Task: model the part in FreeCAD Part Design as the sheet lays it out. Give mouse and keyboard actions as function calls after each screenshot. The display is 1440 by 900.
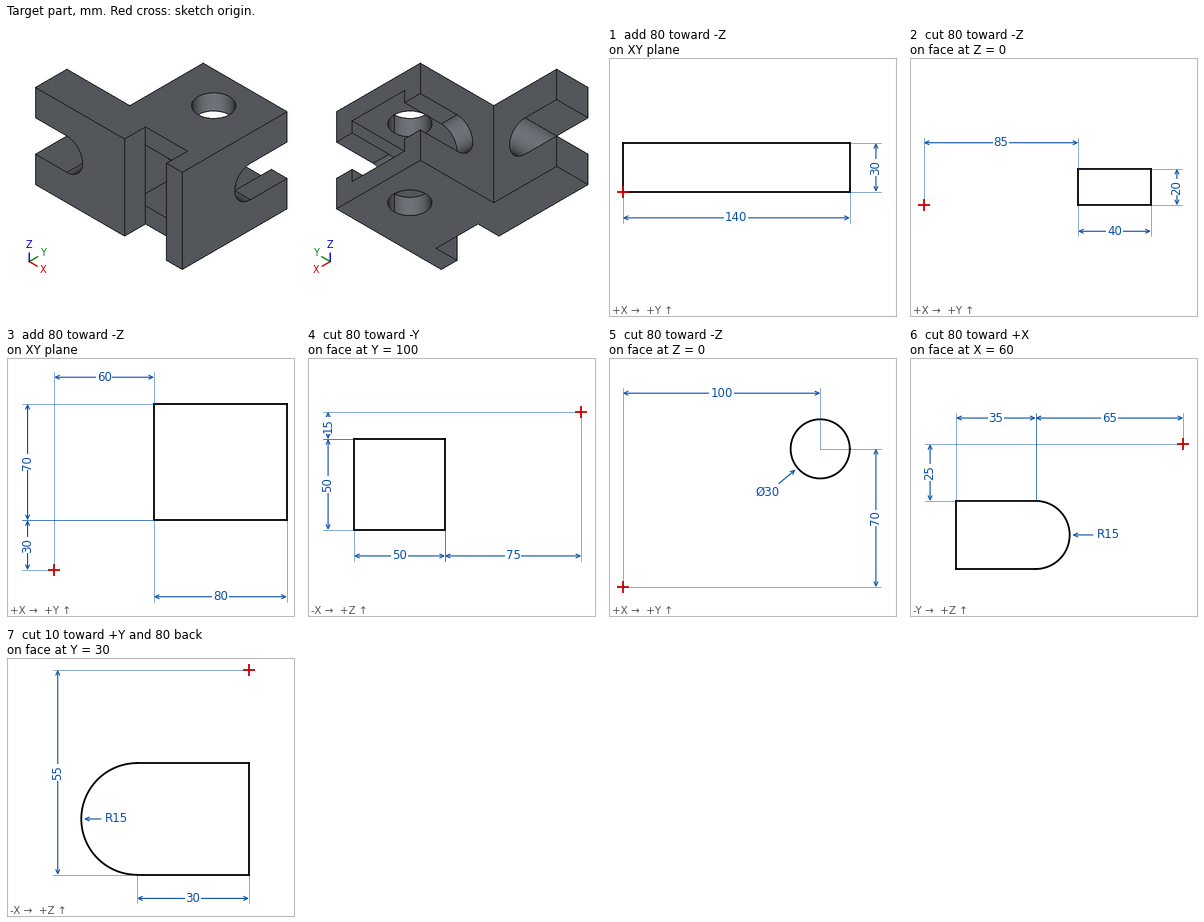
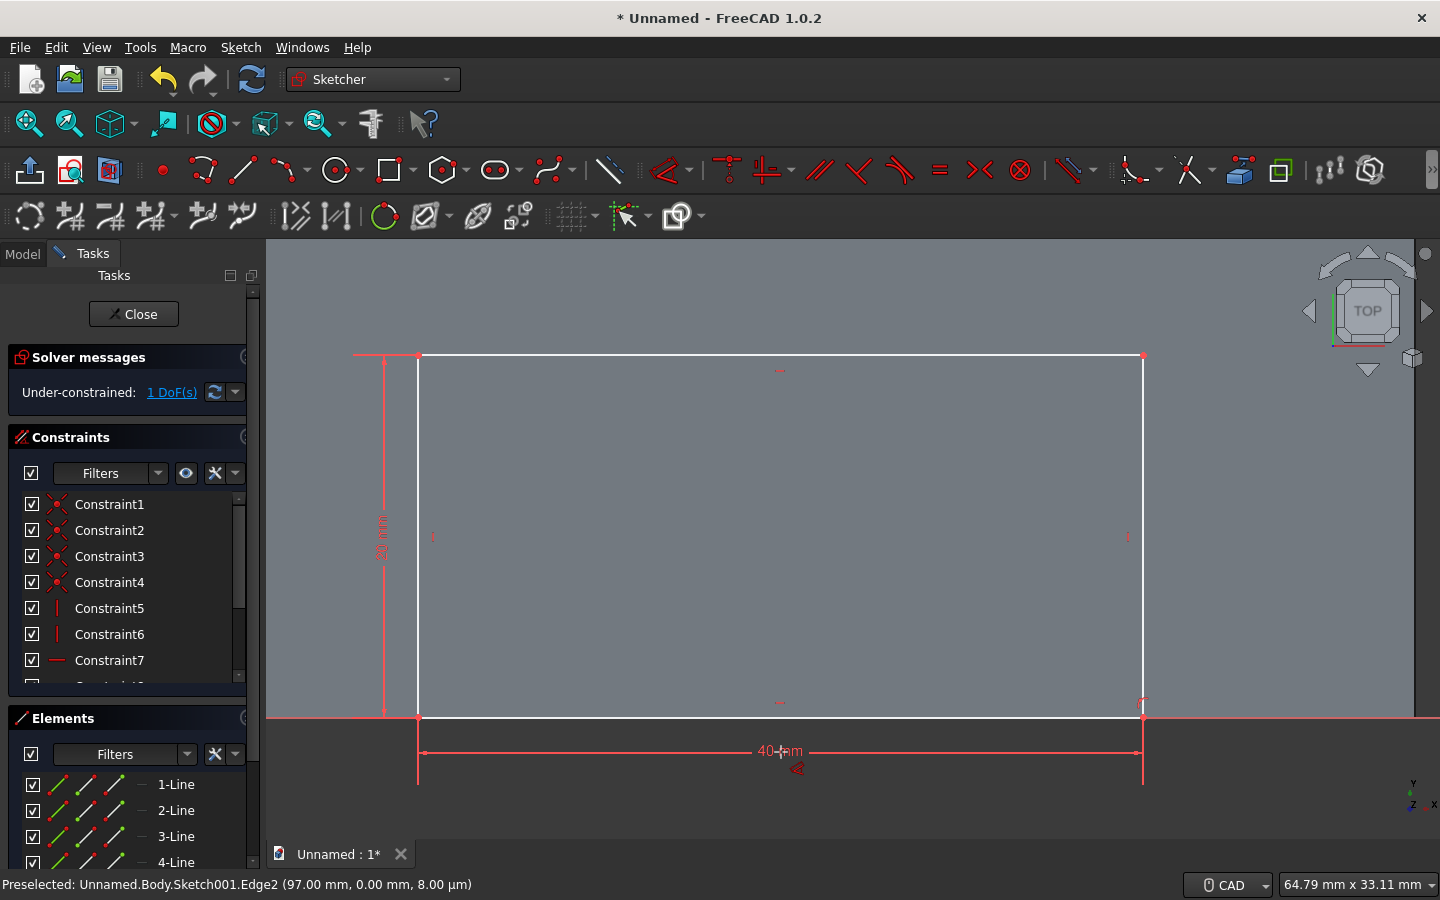
click(418, 355)
click(356, 752)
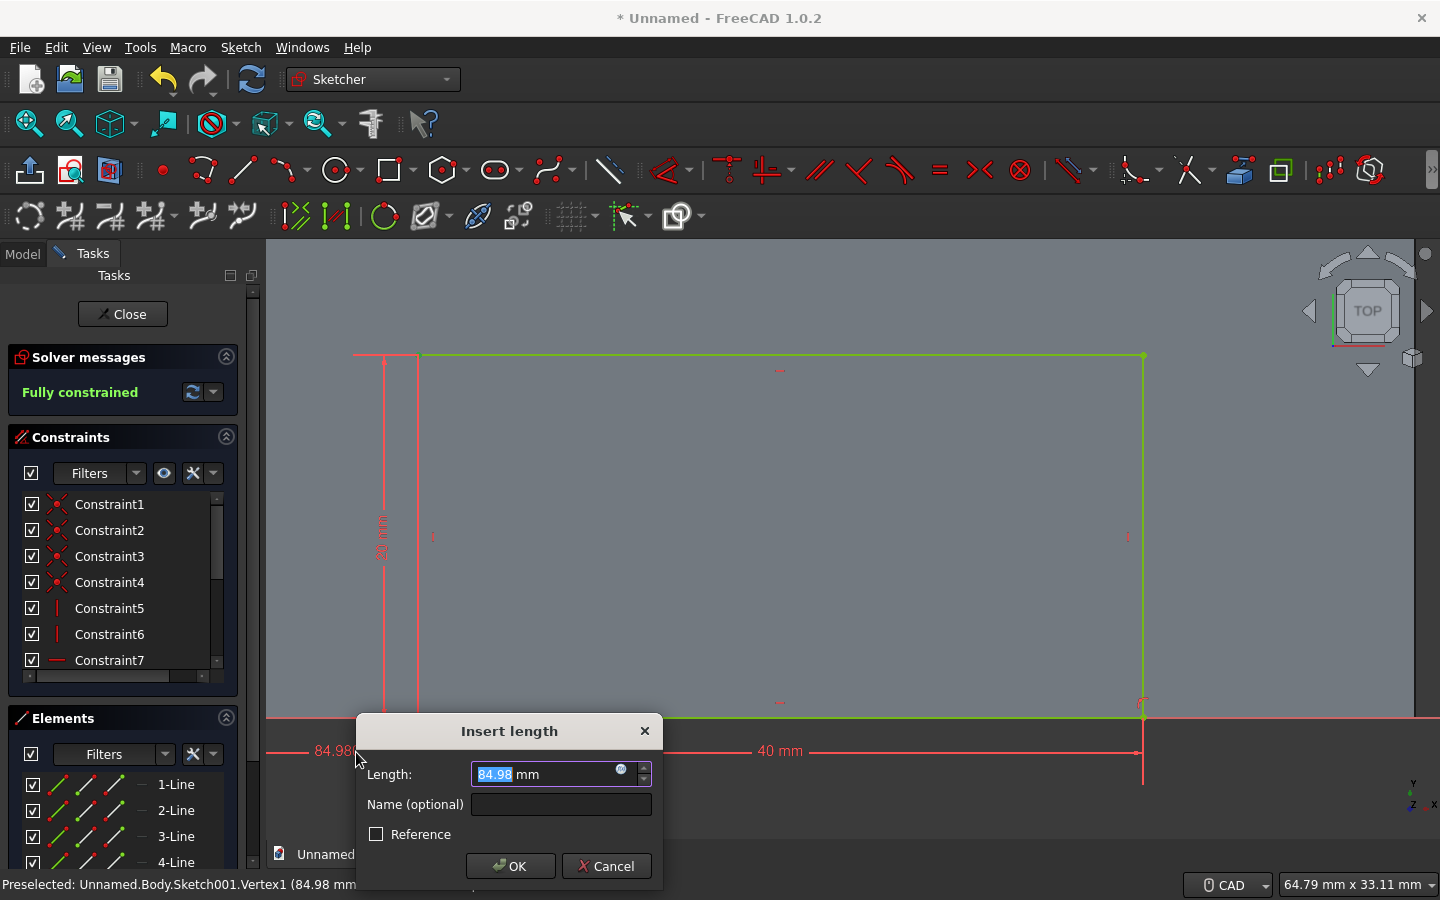
text(85)
key(Return)
key(Escape)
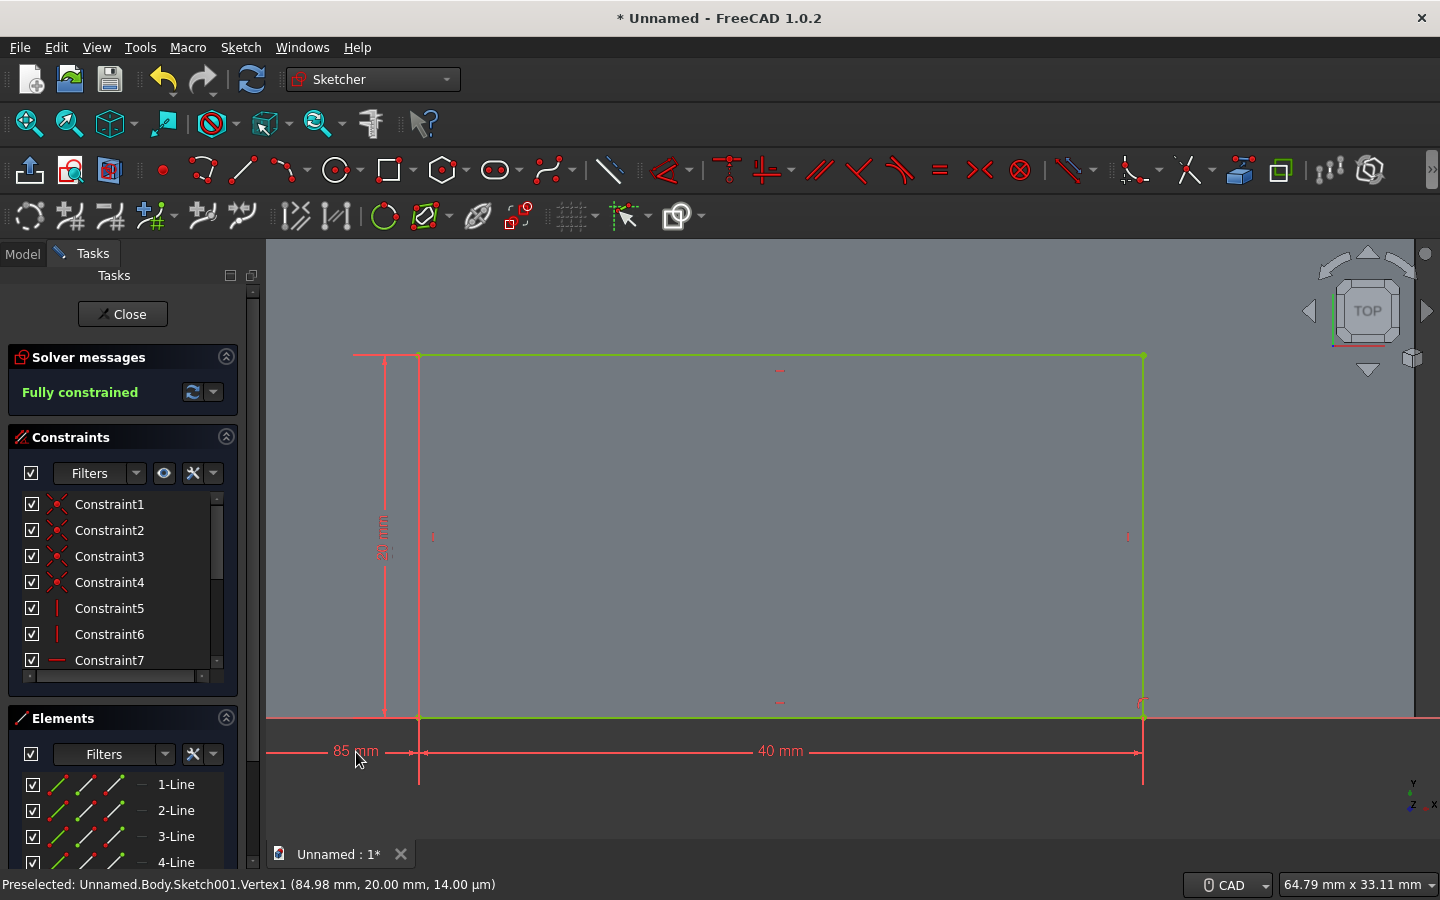
click(123, 314)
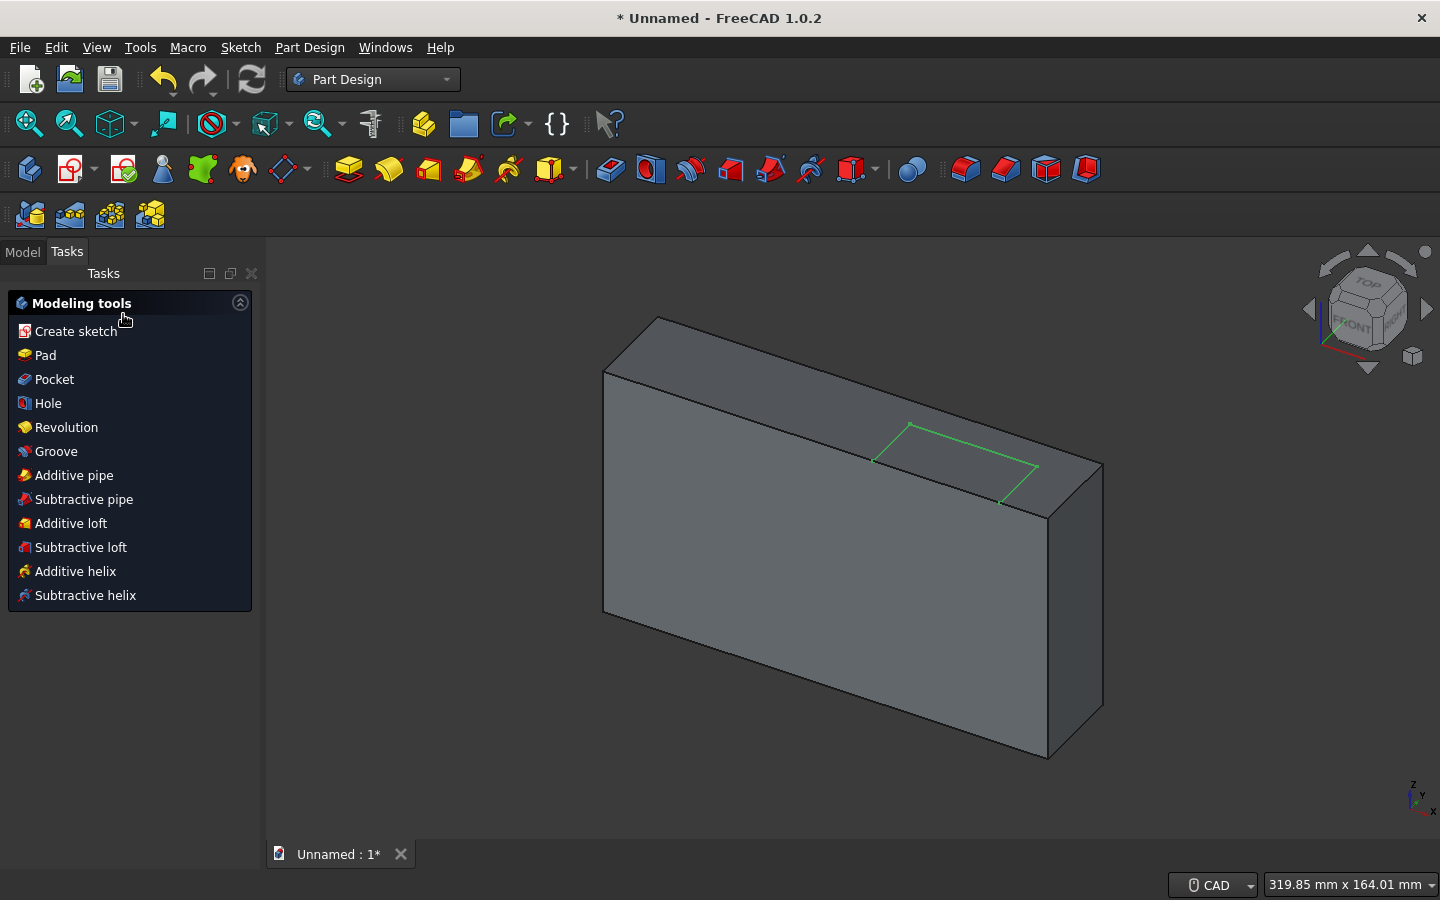
click(612, 170)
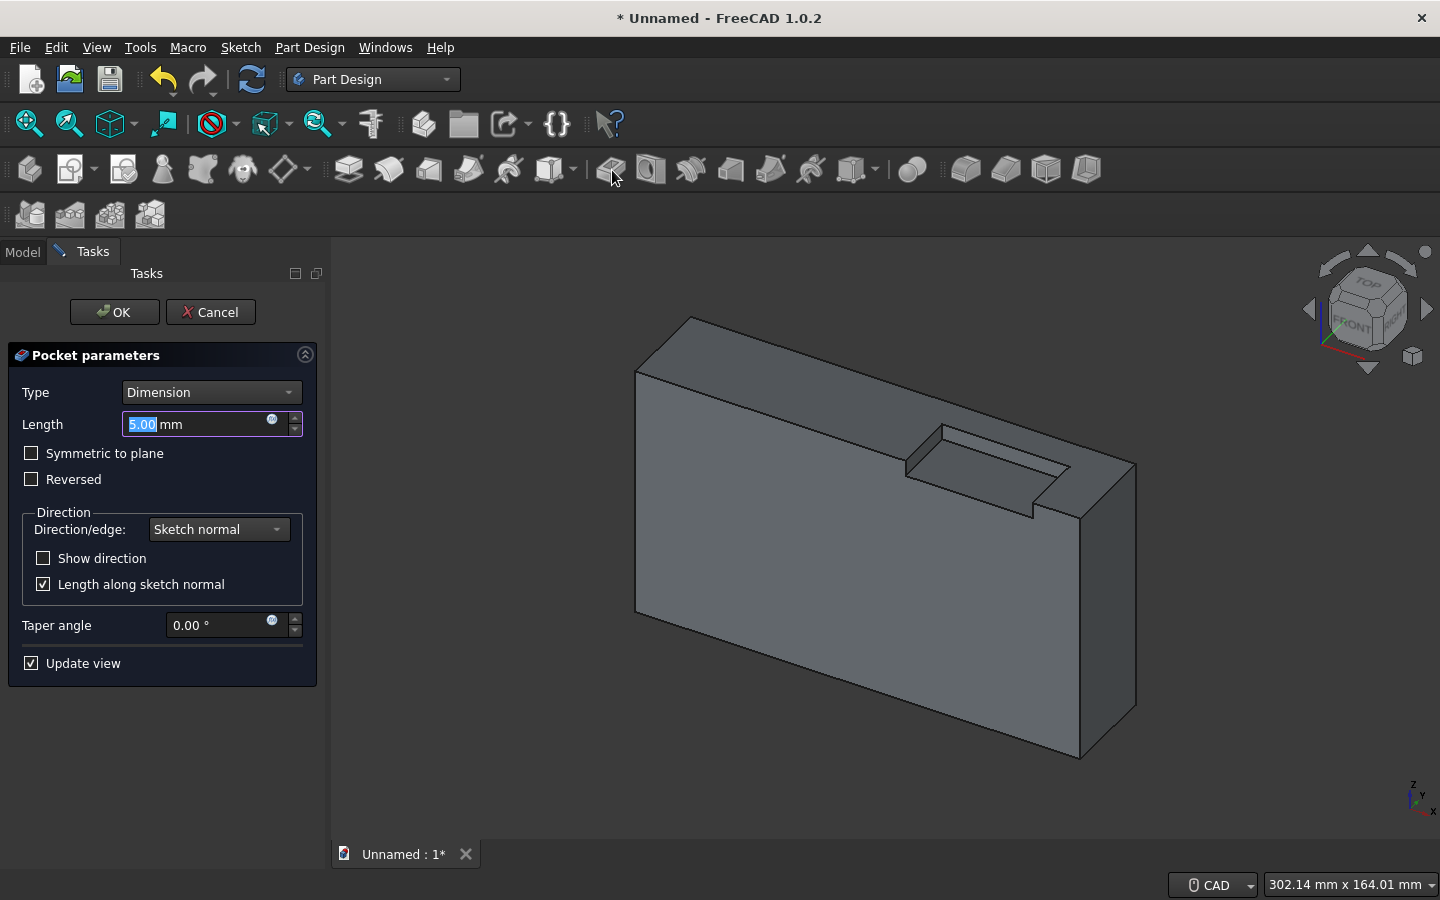
text(80)
key(Tab)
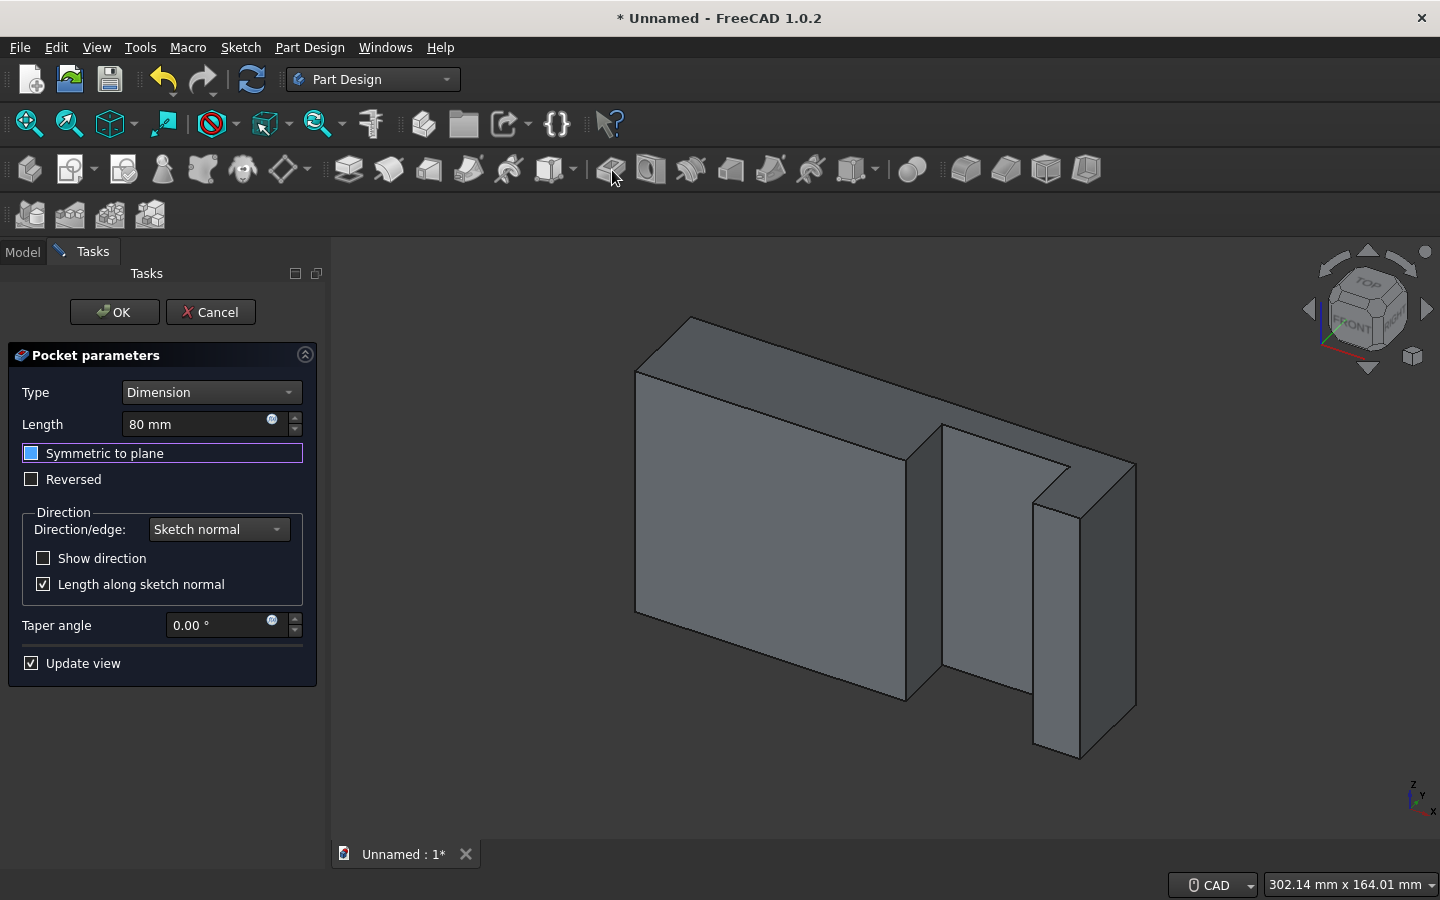
click(115, 312)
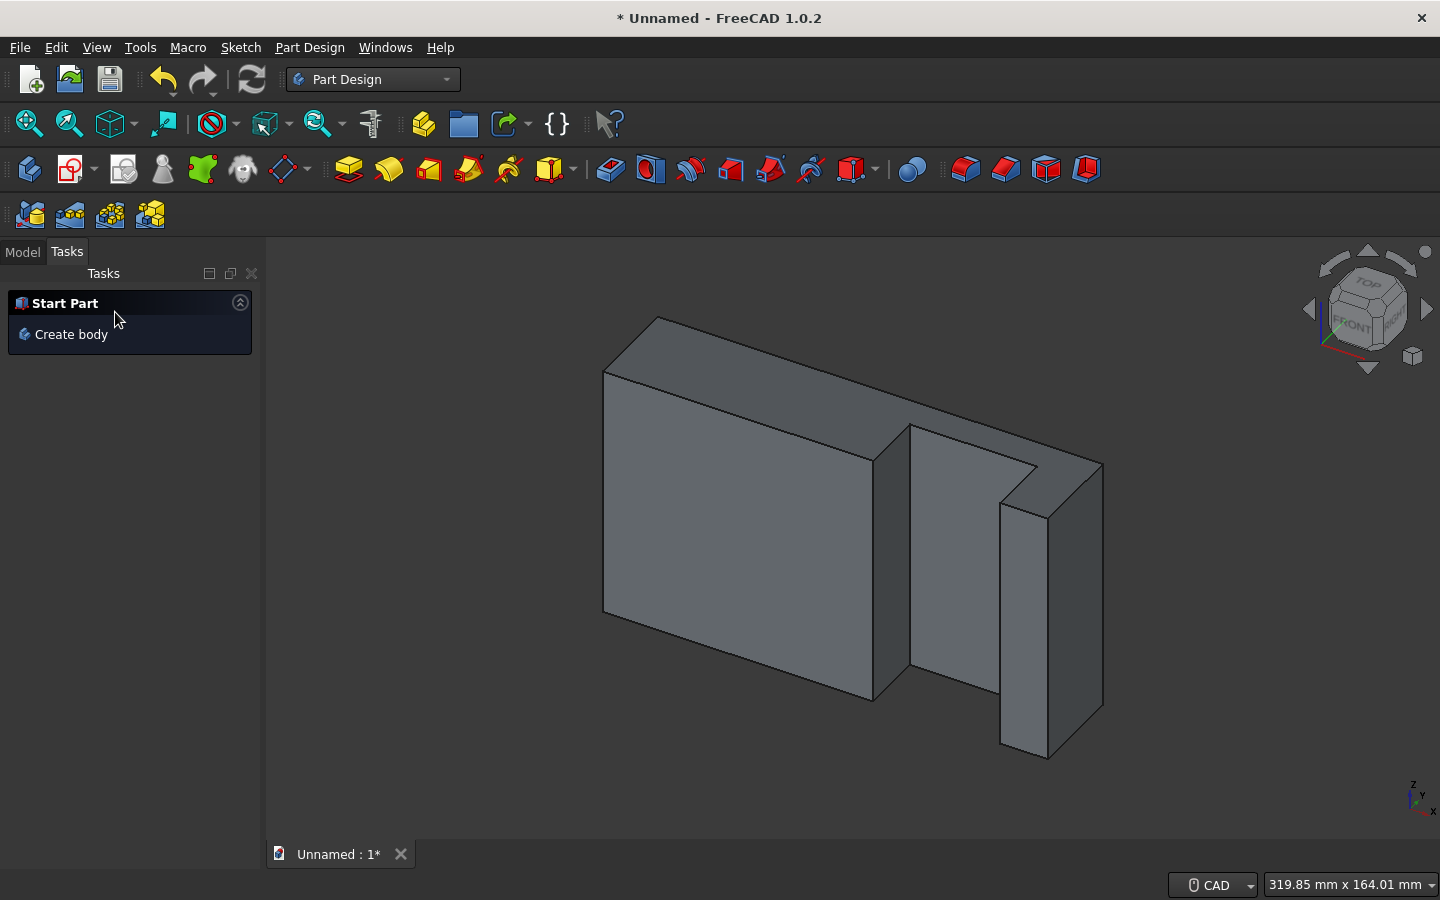
click(70, 170)